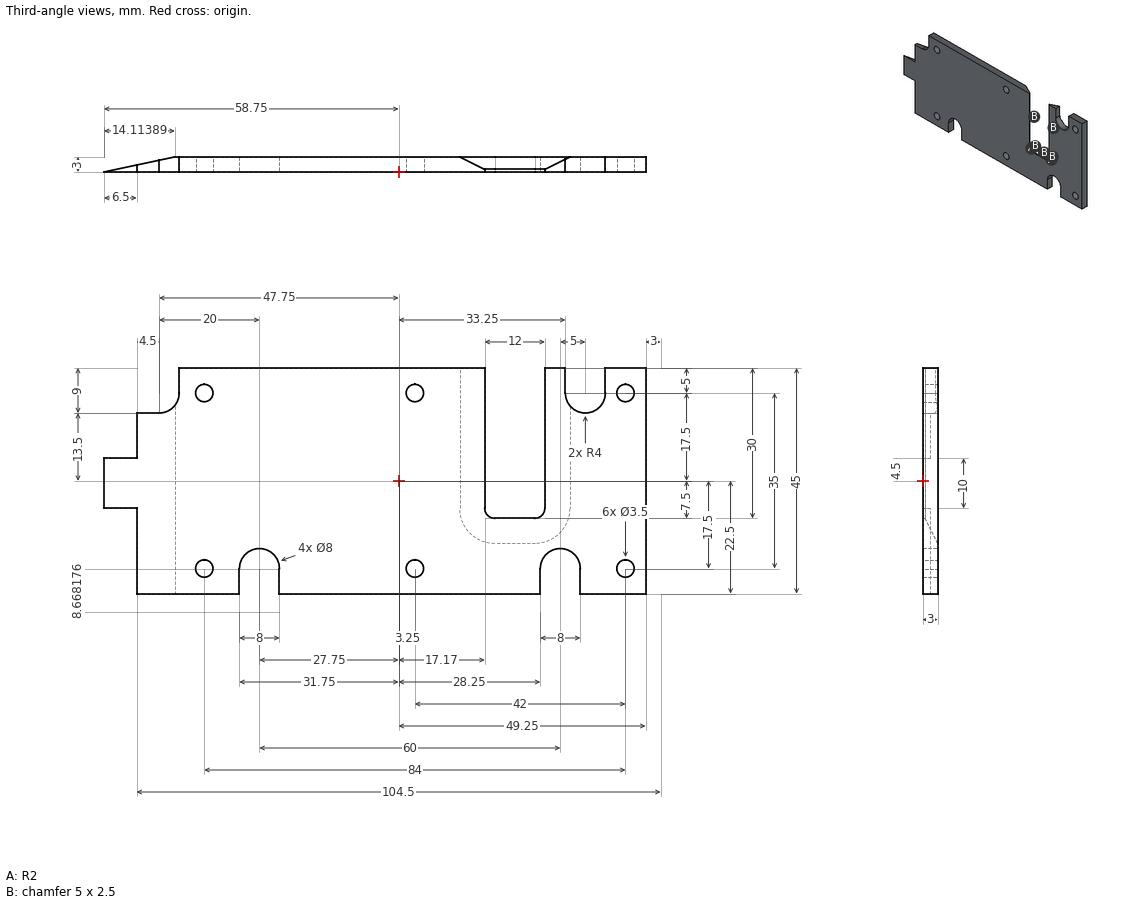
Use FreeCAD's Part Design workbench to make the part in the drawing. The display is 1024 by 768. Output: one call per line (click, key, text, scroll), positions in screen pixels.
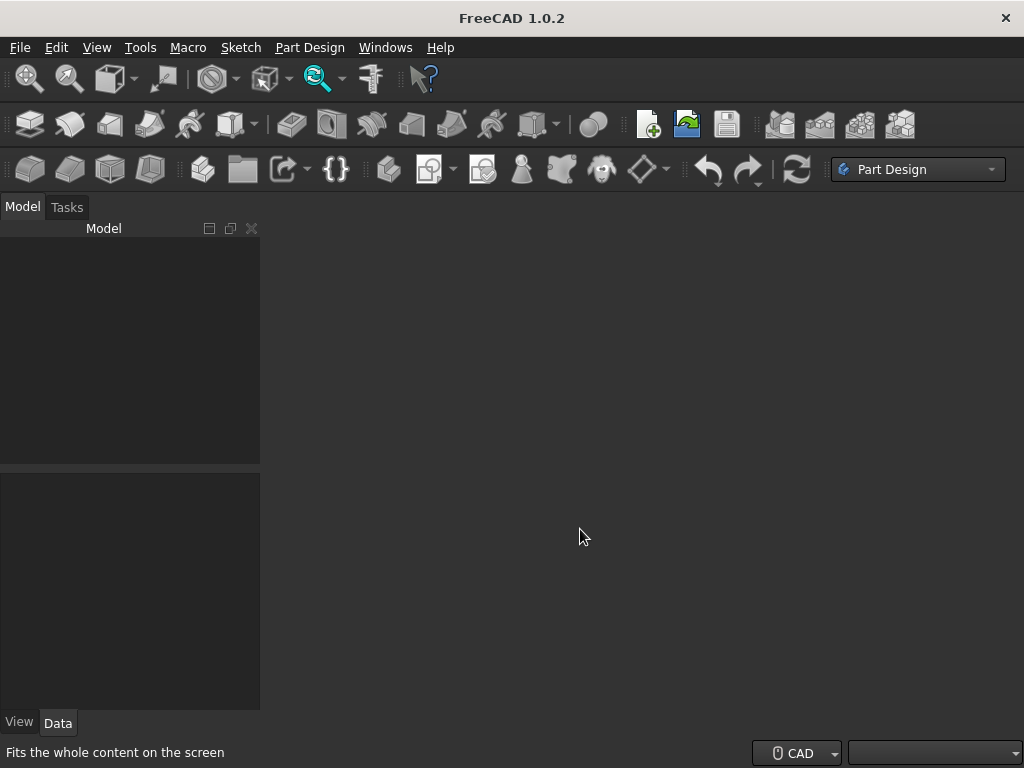
key(ctrl+n)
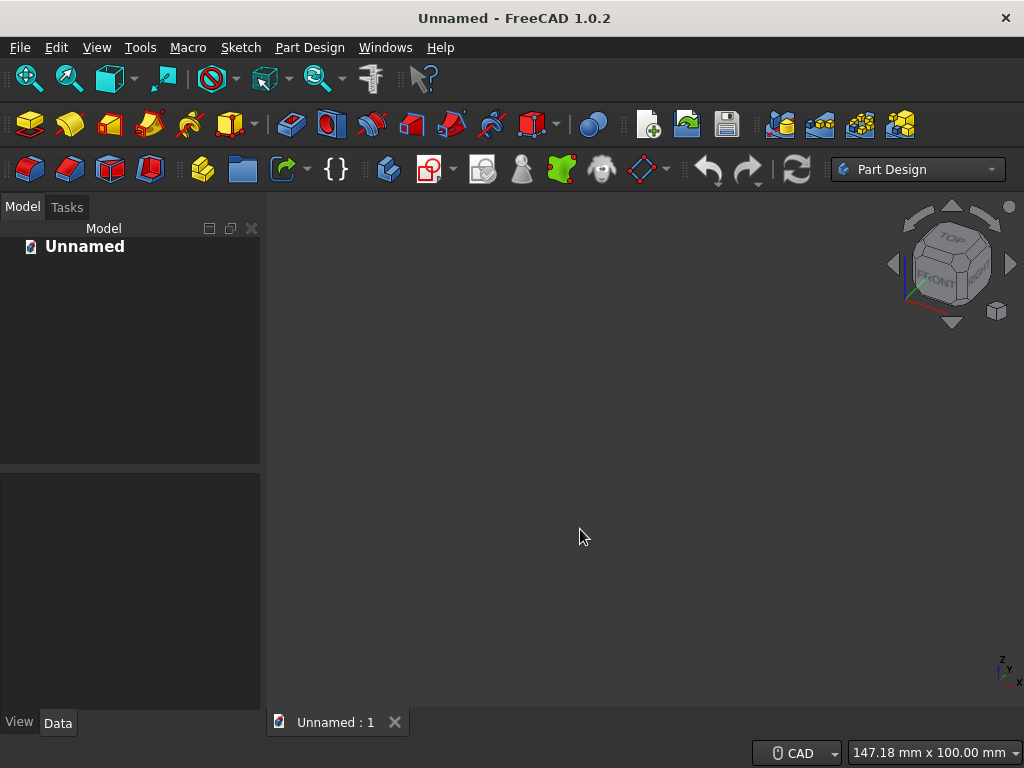
click(430, 170)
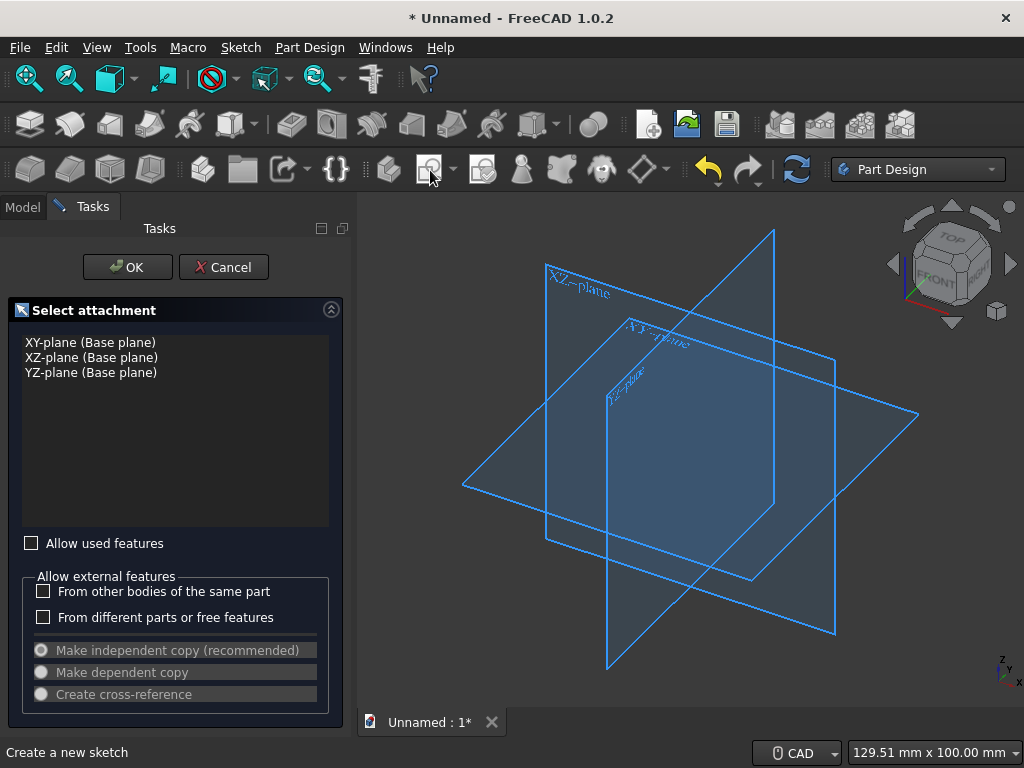
click(82, 358)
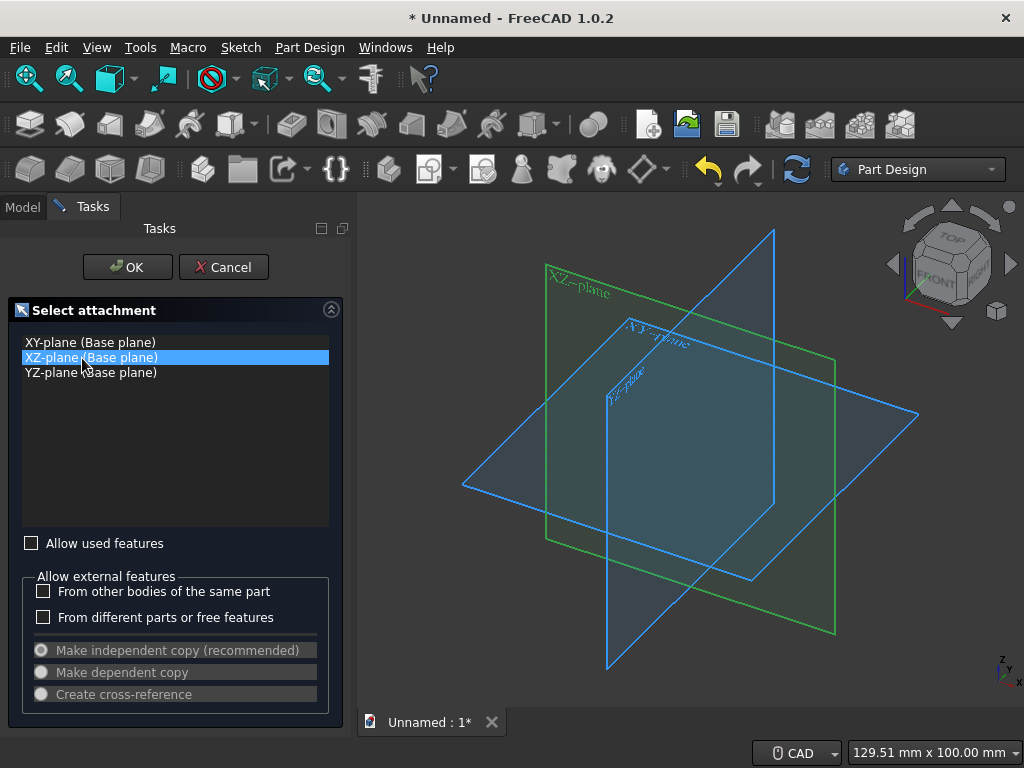
click(128, 267)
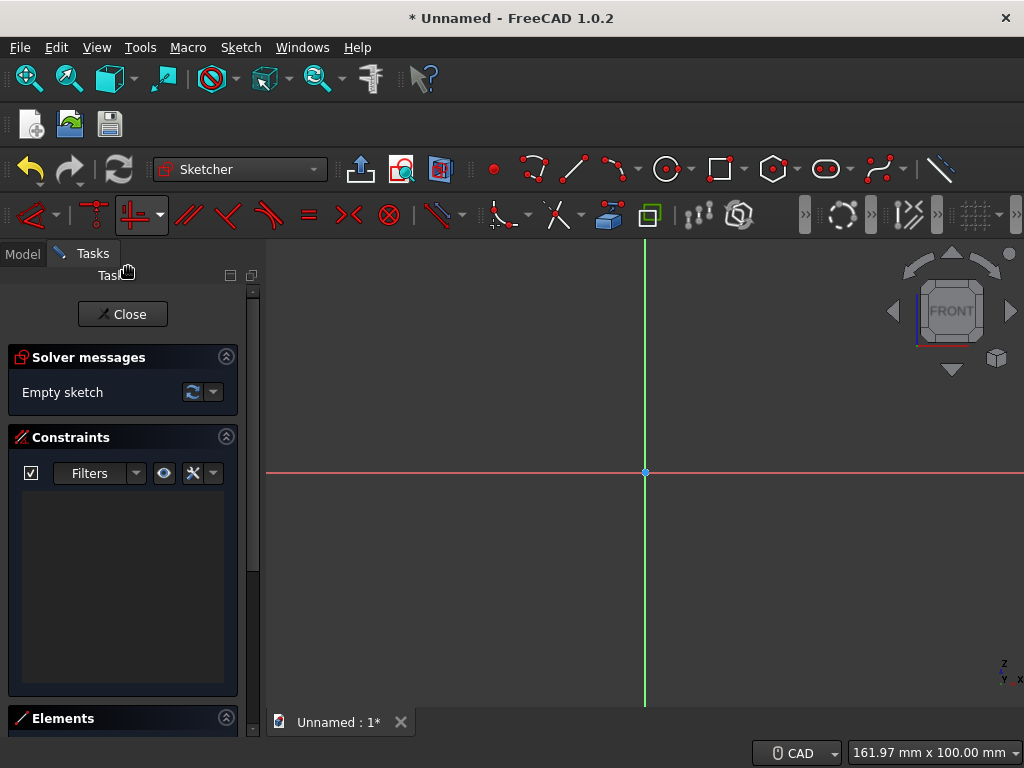
scroll(294, 473, down, 1)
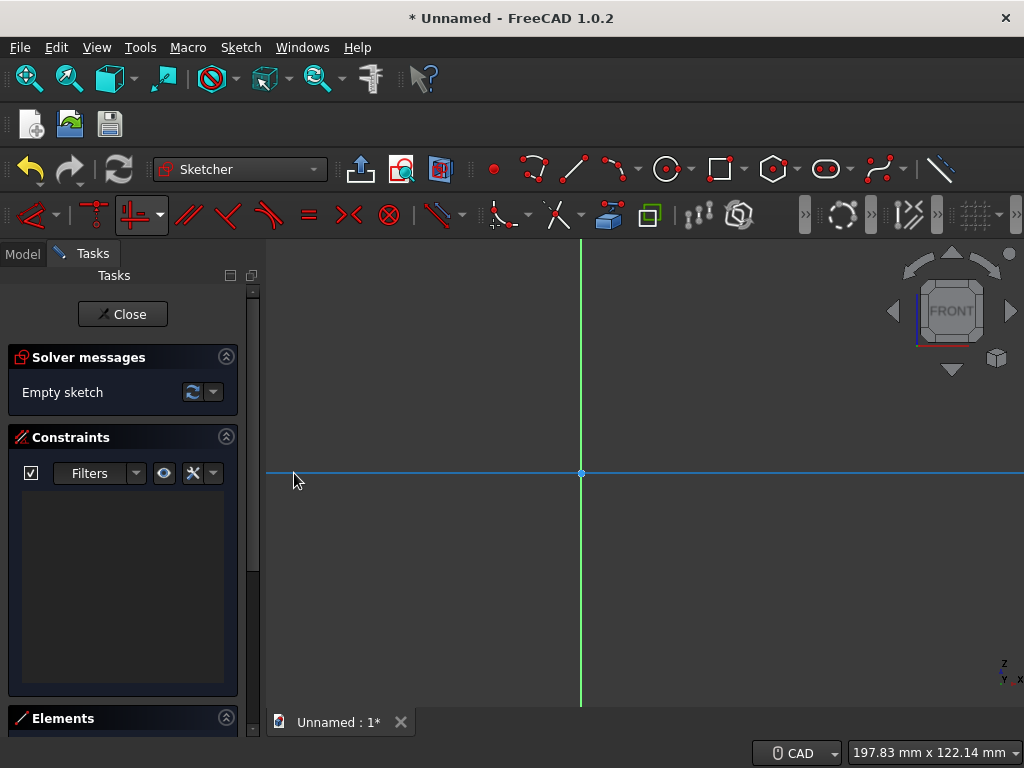
key(g)
key(v)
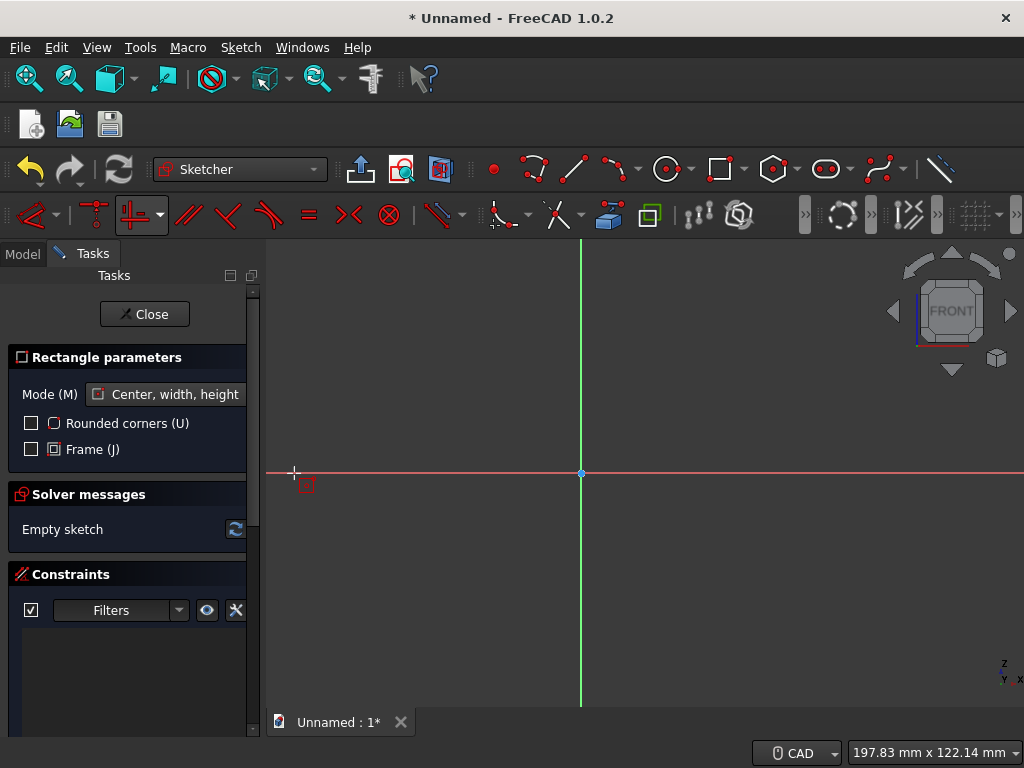
click(581, 473)
move(782, 387)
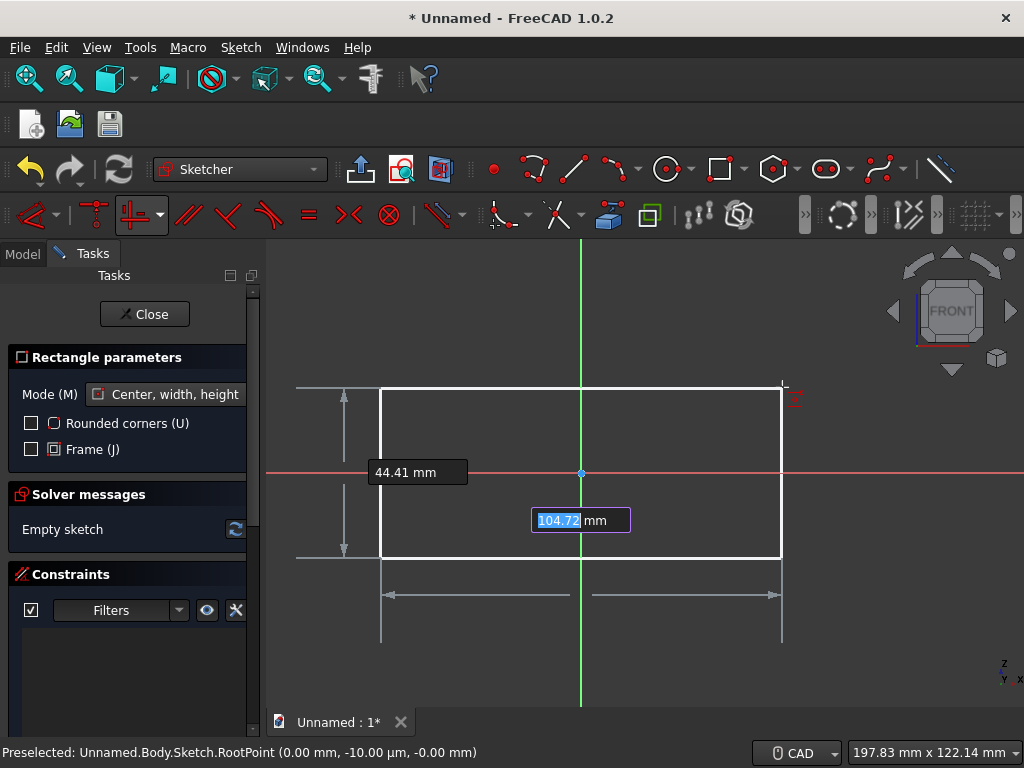
text(104.5)
key(Tab)
text(45)
key(Return)
key(Escape)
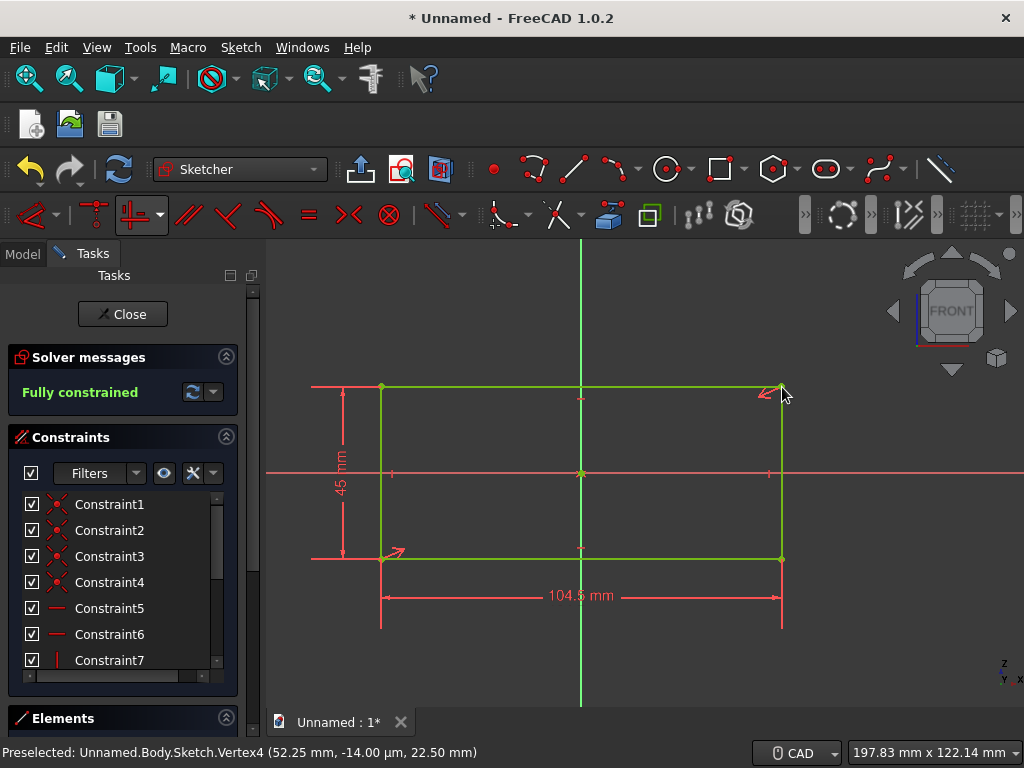
click(123, 314)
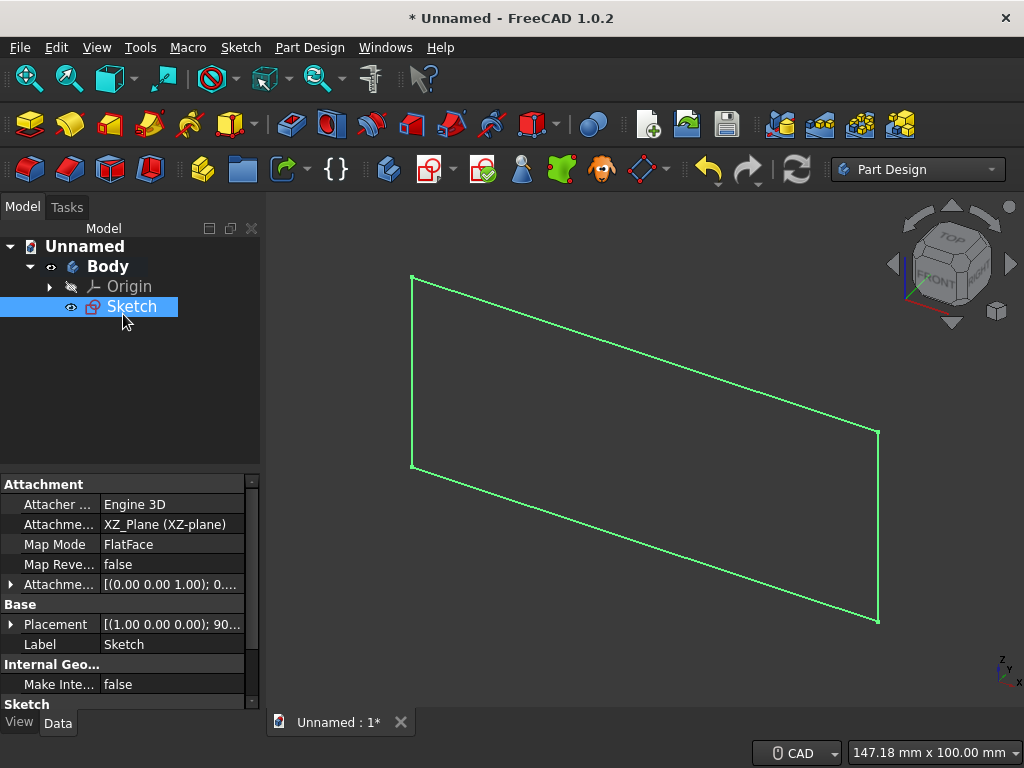
click(30, 124)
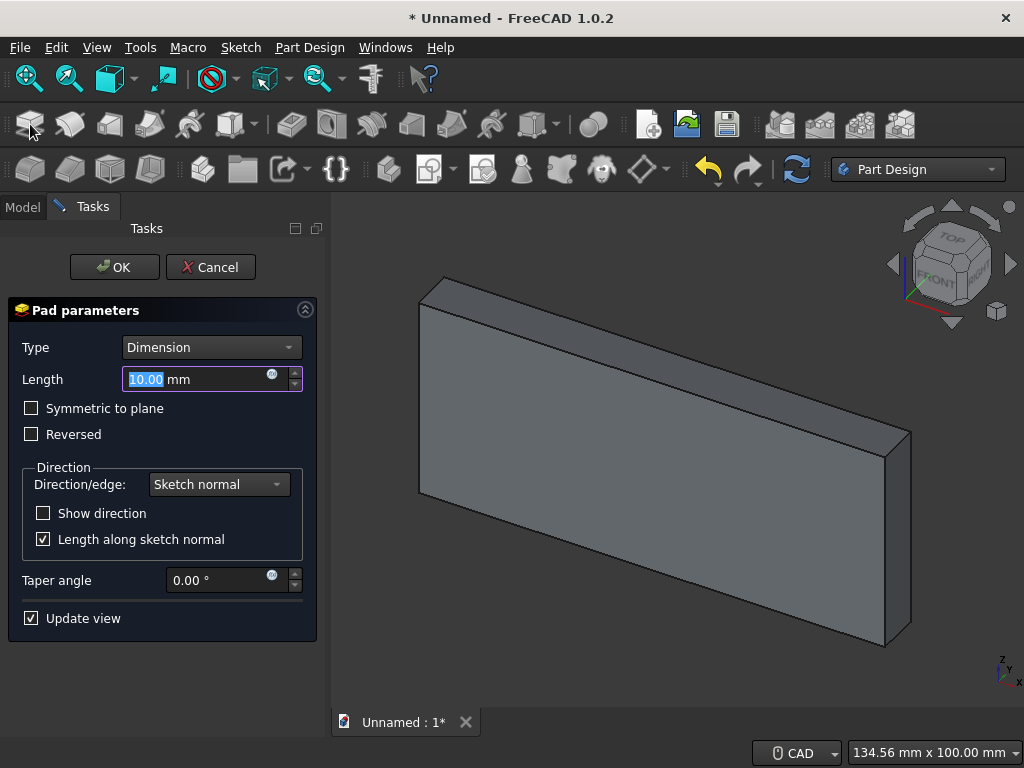
text(3)
key(Tab)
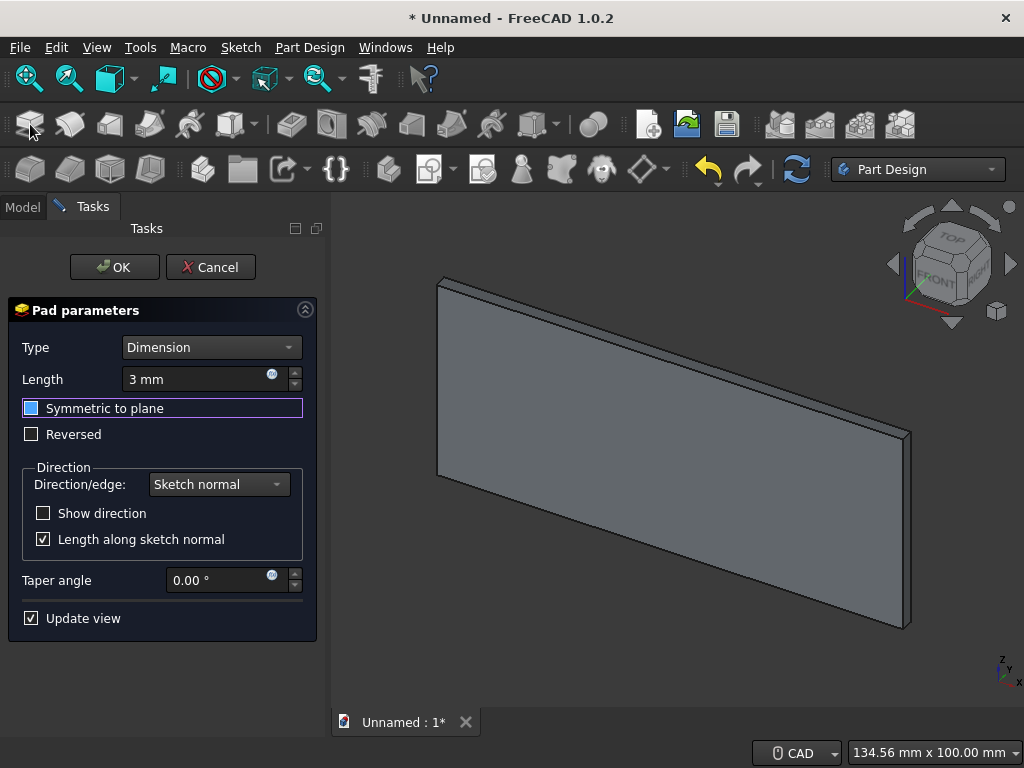
click(30, 434)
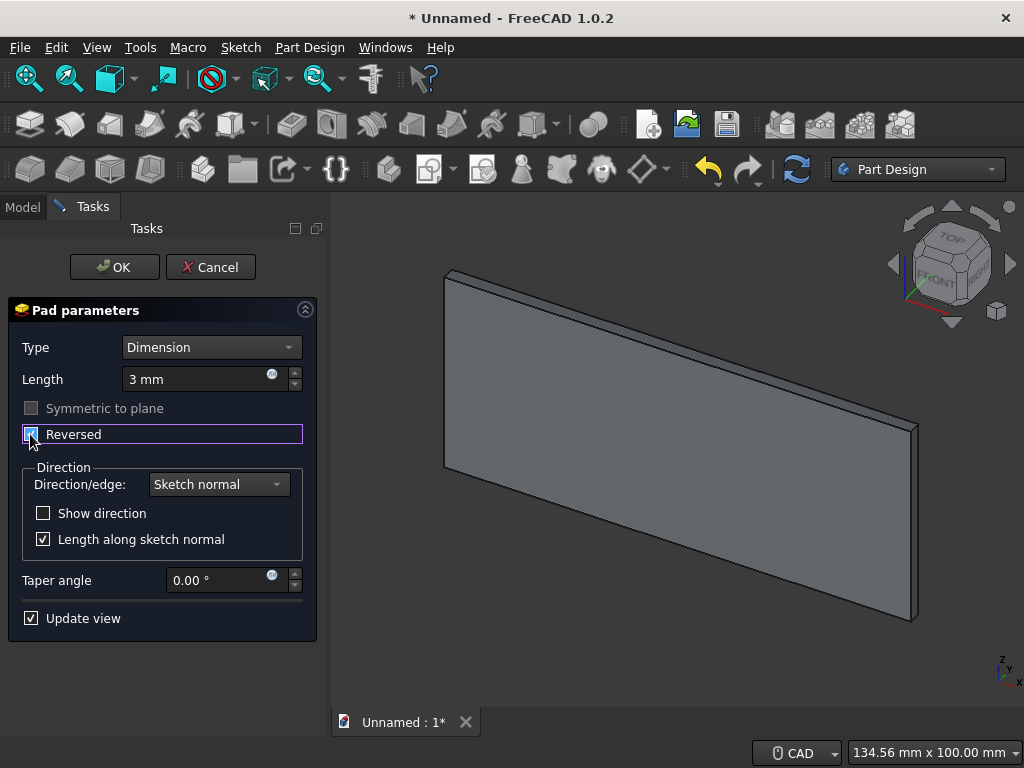
click(115, 267)